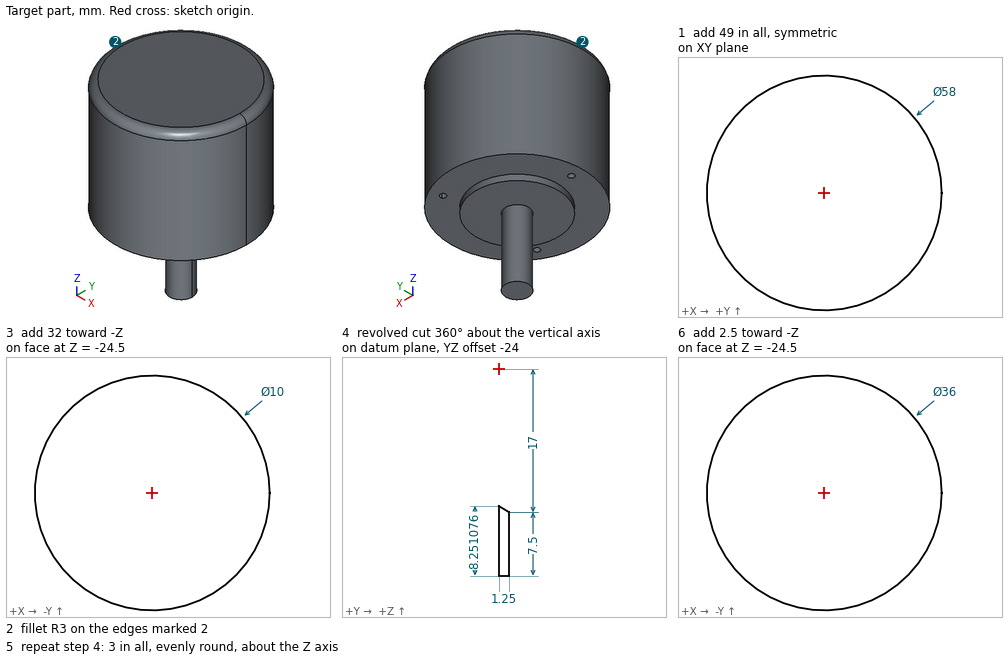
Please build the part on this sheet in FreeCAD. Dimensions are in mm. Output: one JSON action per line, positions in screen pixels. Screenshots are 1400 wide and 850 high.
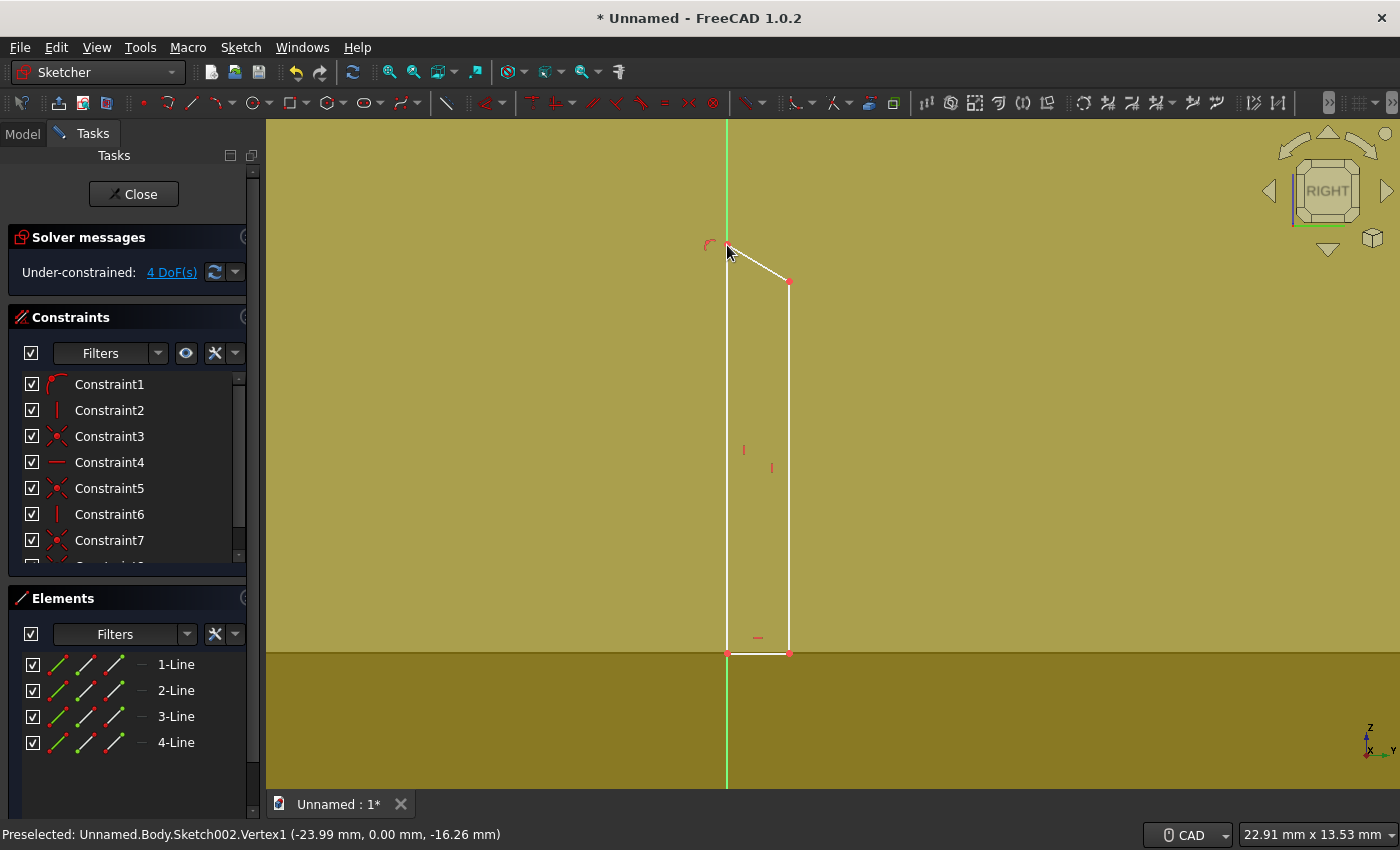
{"action": "left_click", "coordinate": [486, 104]}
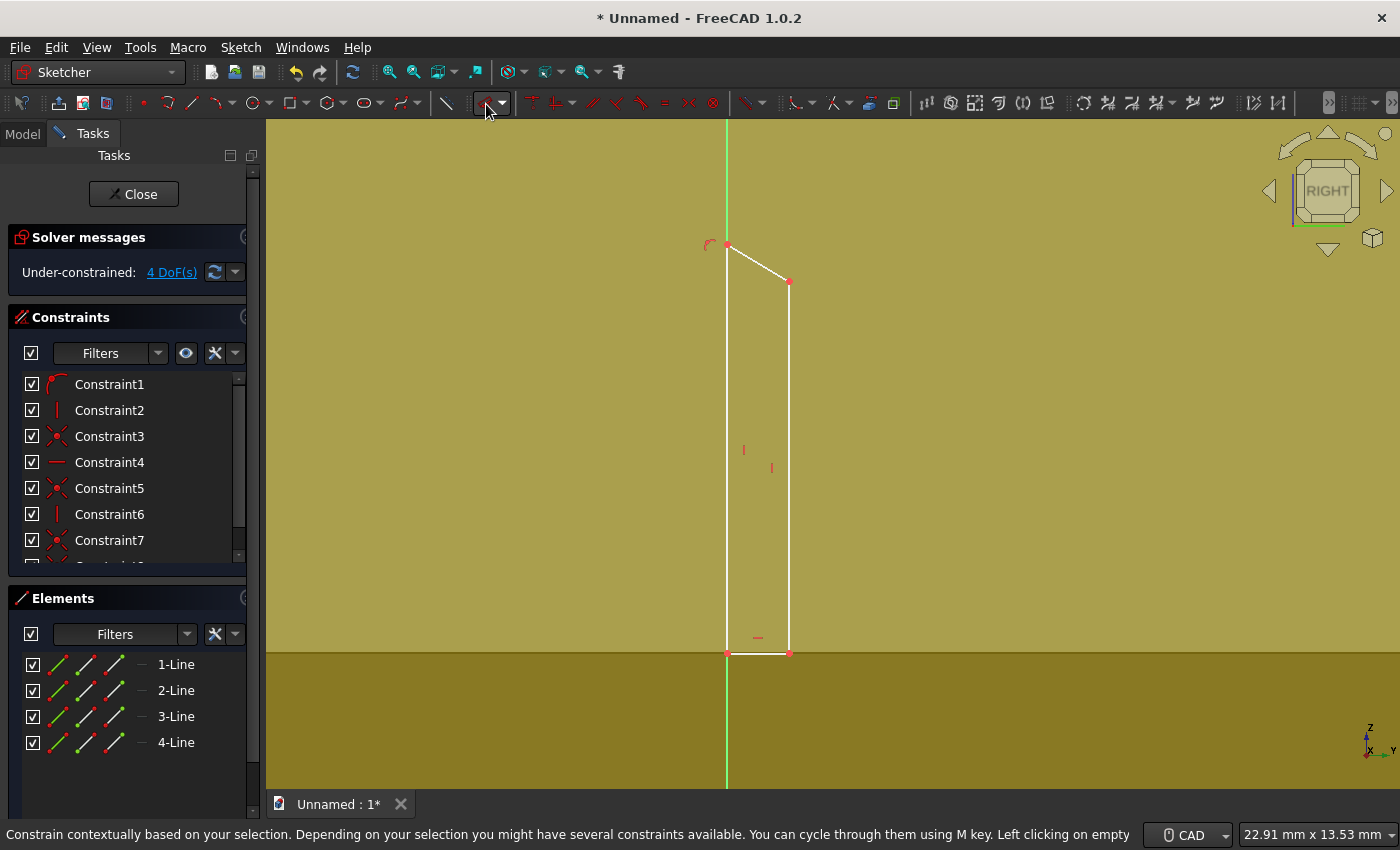
{"action": "left_click", "coordinate": [789, 542]}
{"action": "left_click", "coordinate": [823, 468]}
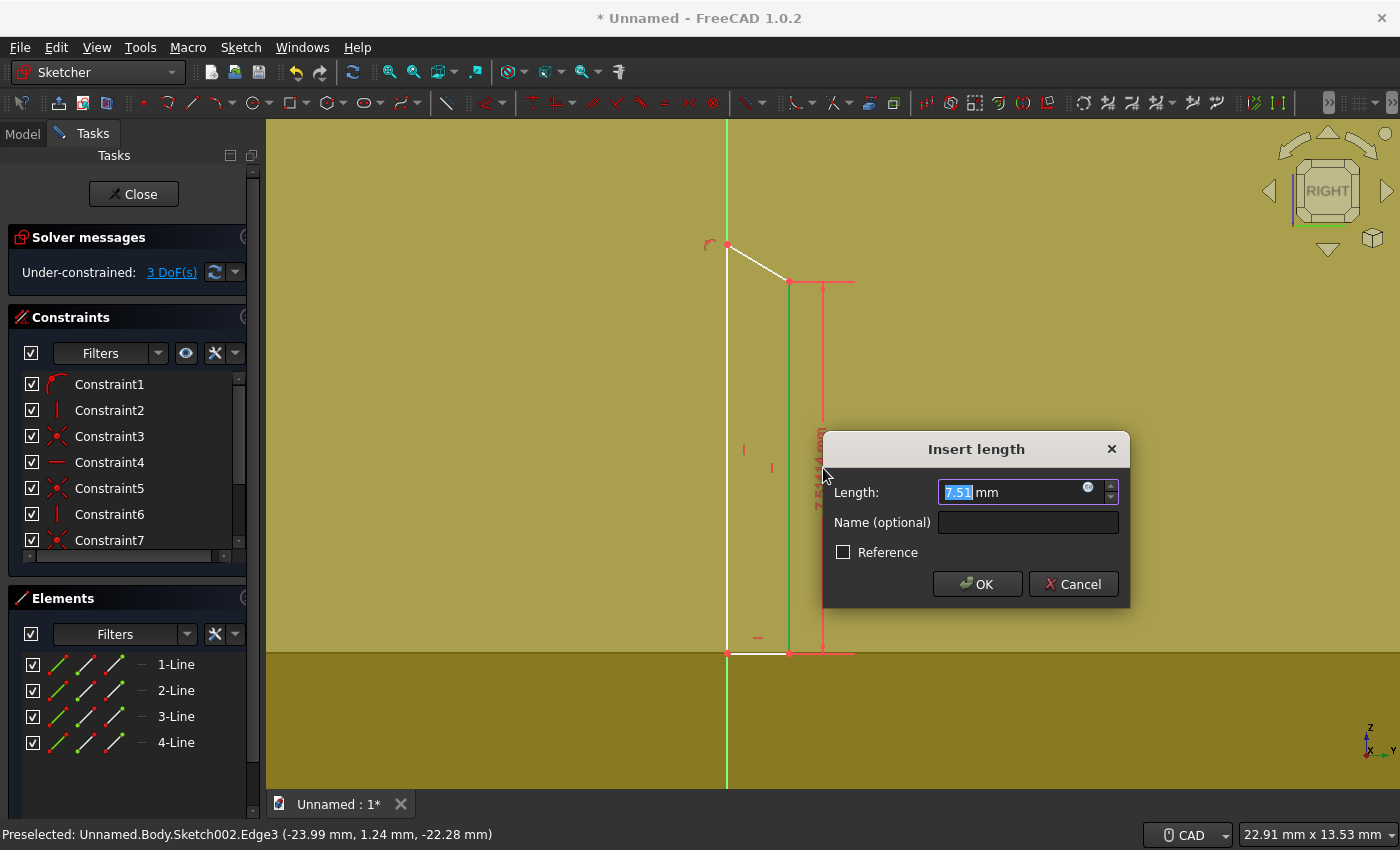
{"action": "type", "text": "7.5"}
{"action": "key", "text": "Return"}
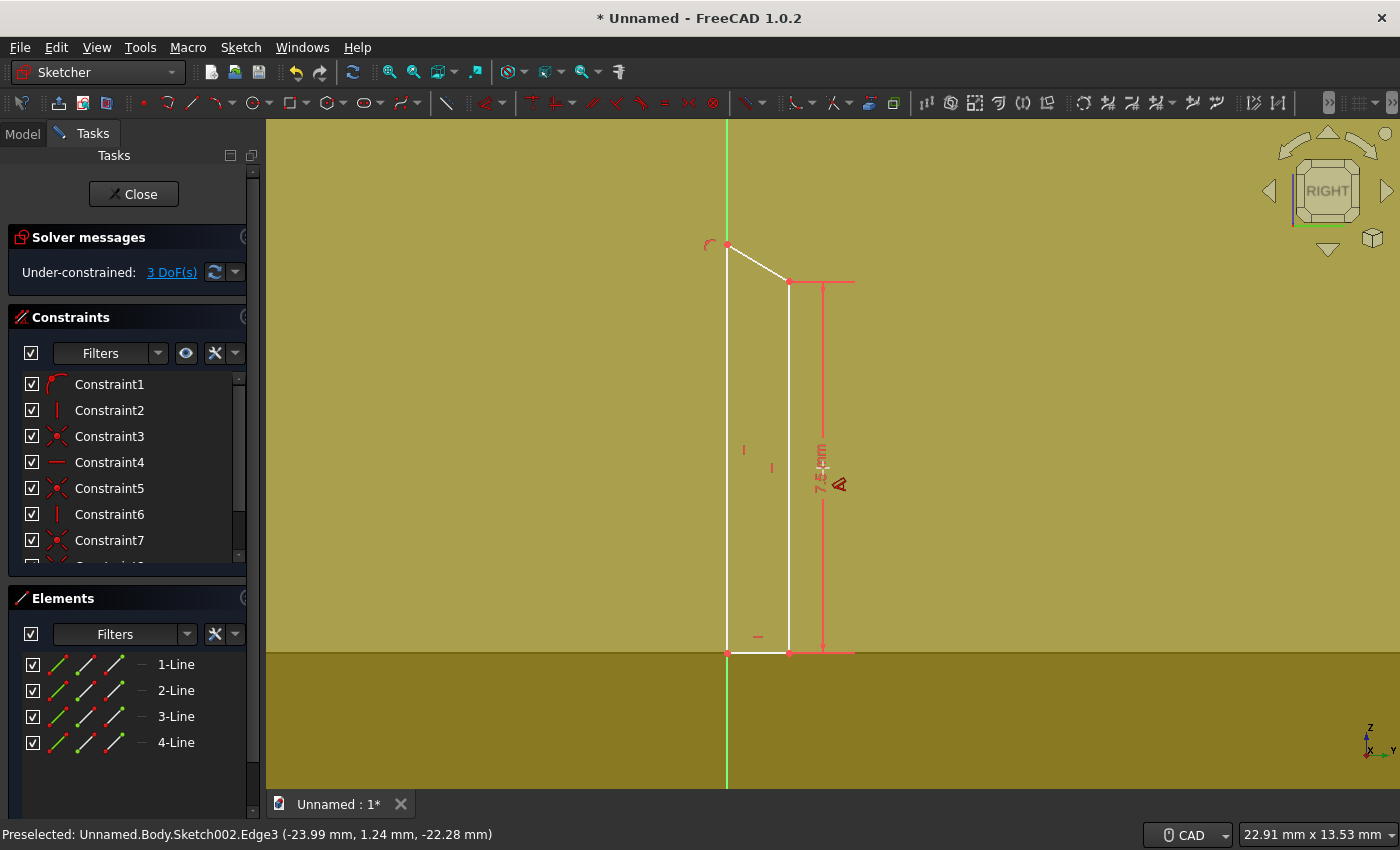
{"action": "left_click", "coordinate": [789, 282]}
{"action": "left_click", "coordinate": [693, 215]}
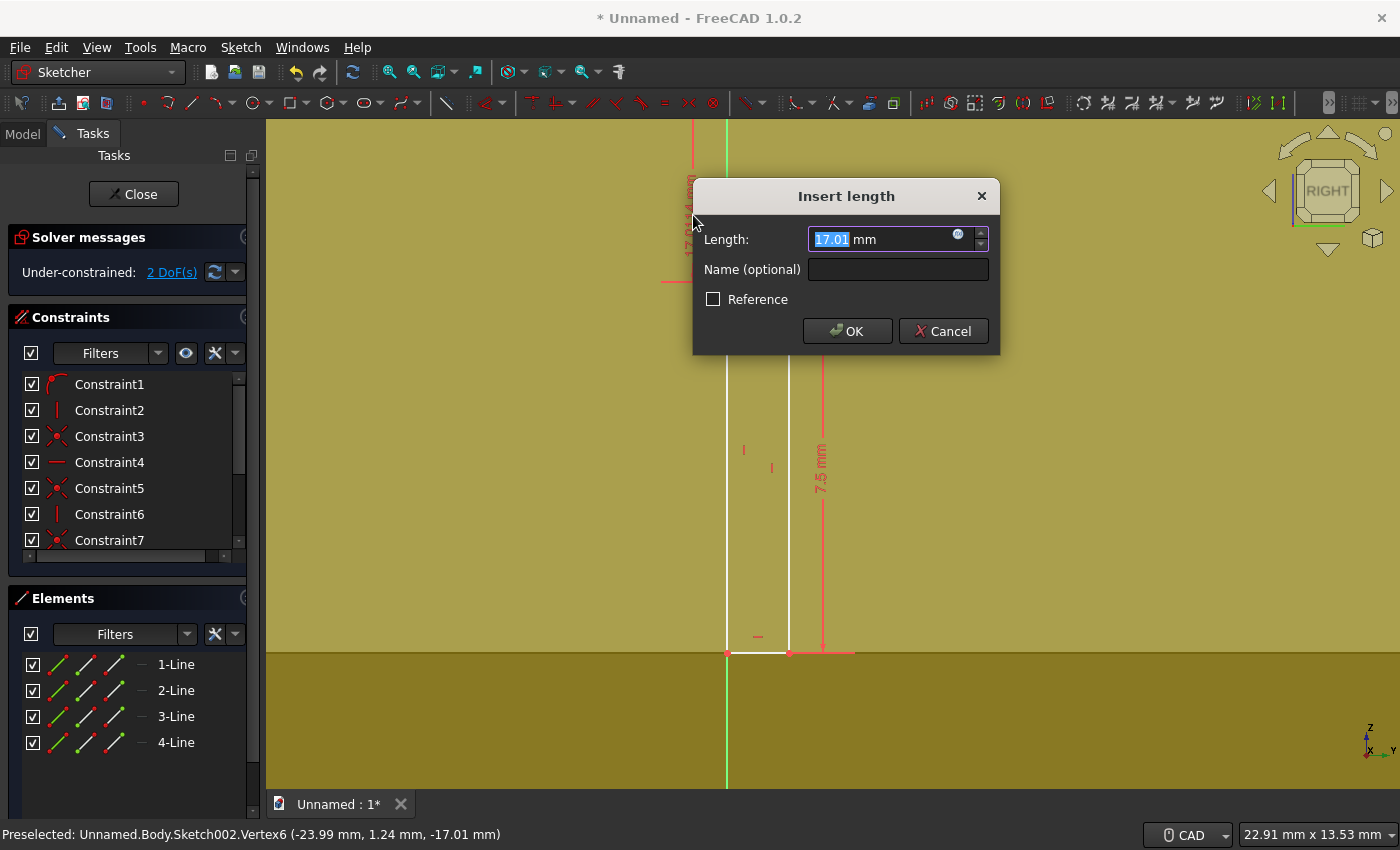
{"action": "type", "text": "17"}
{"action": "key", "text": "Return"}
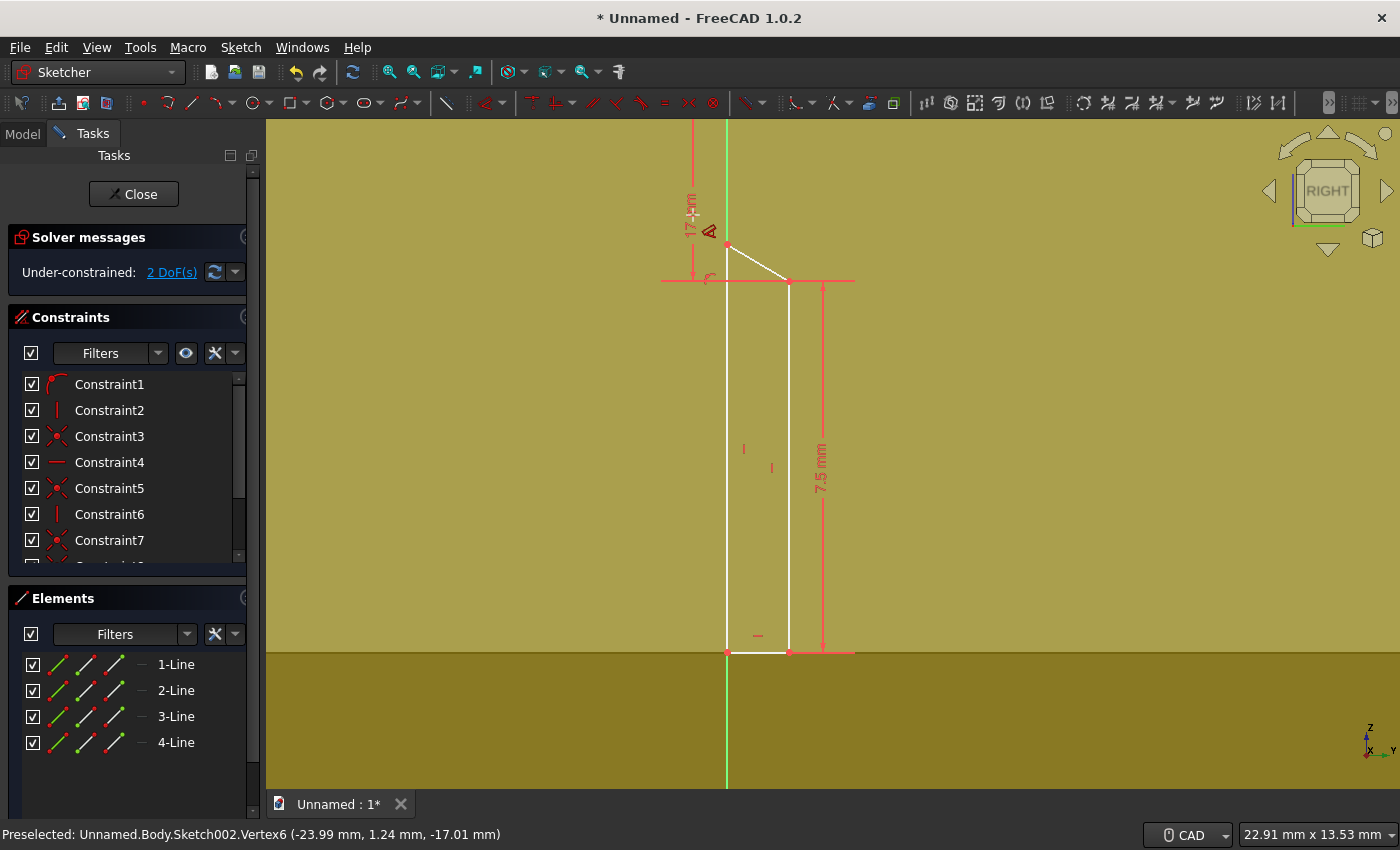
{"action": "left_click", "coordinate": [746, 653]}
{"action": "left_click", "coordinate": [758, 687]}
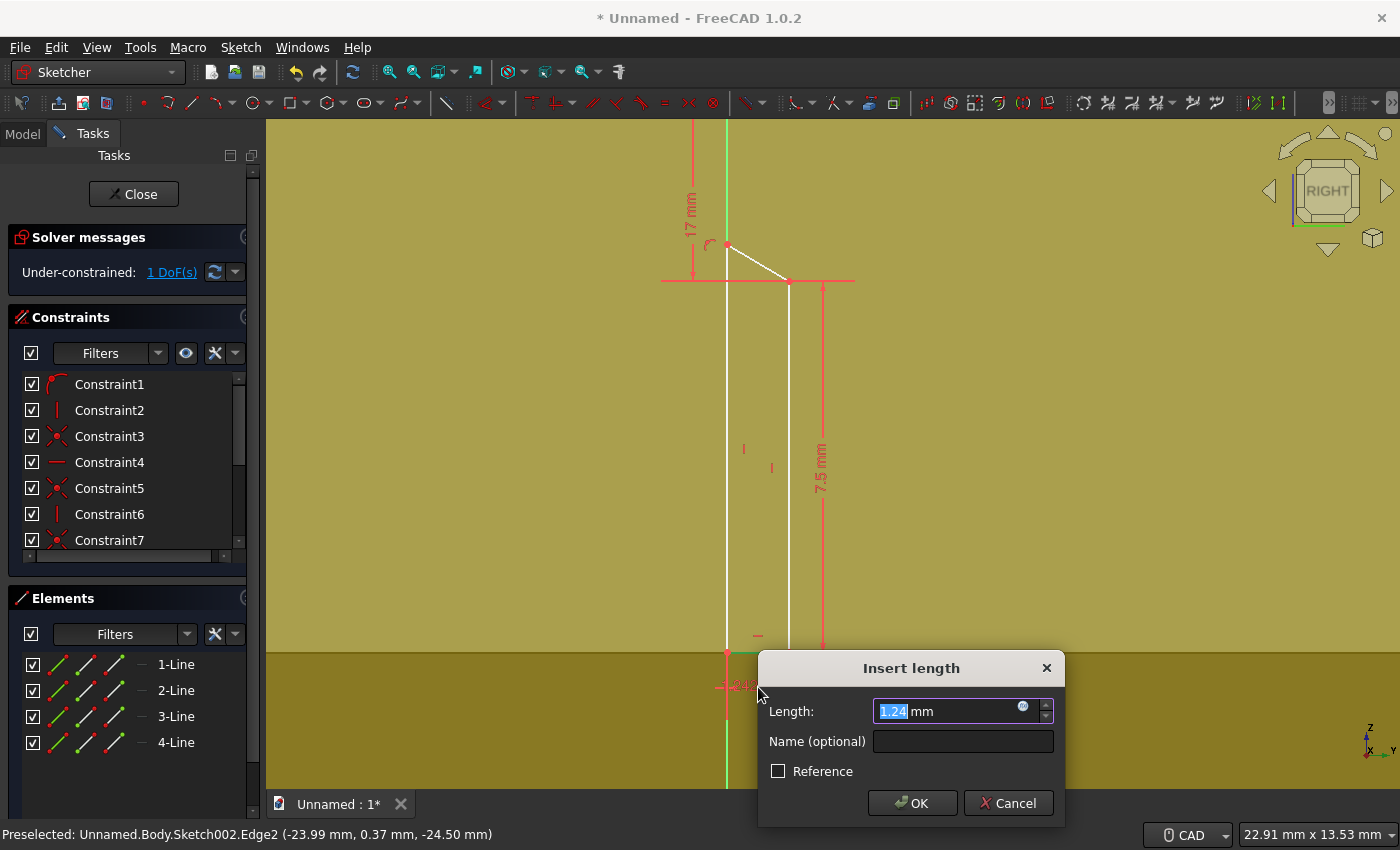
{"action": "type", "text": "1.25"}
{"action": "key", "text": "Return"}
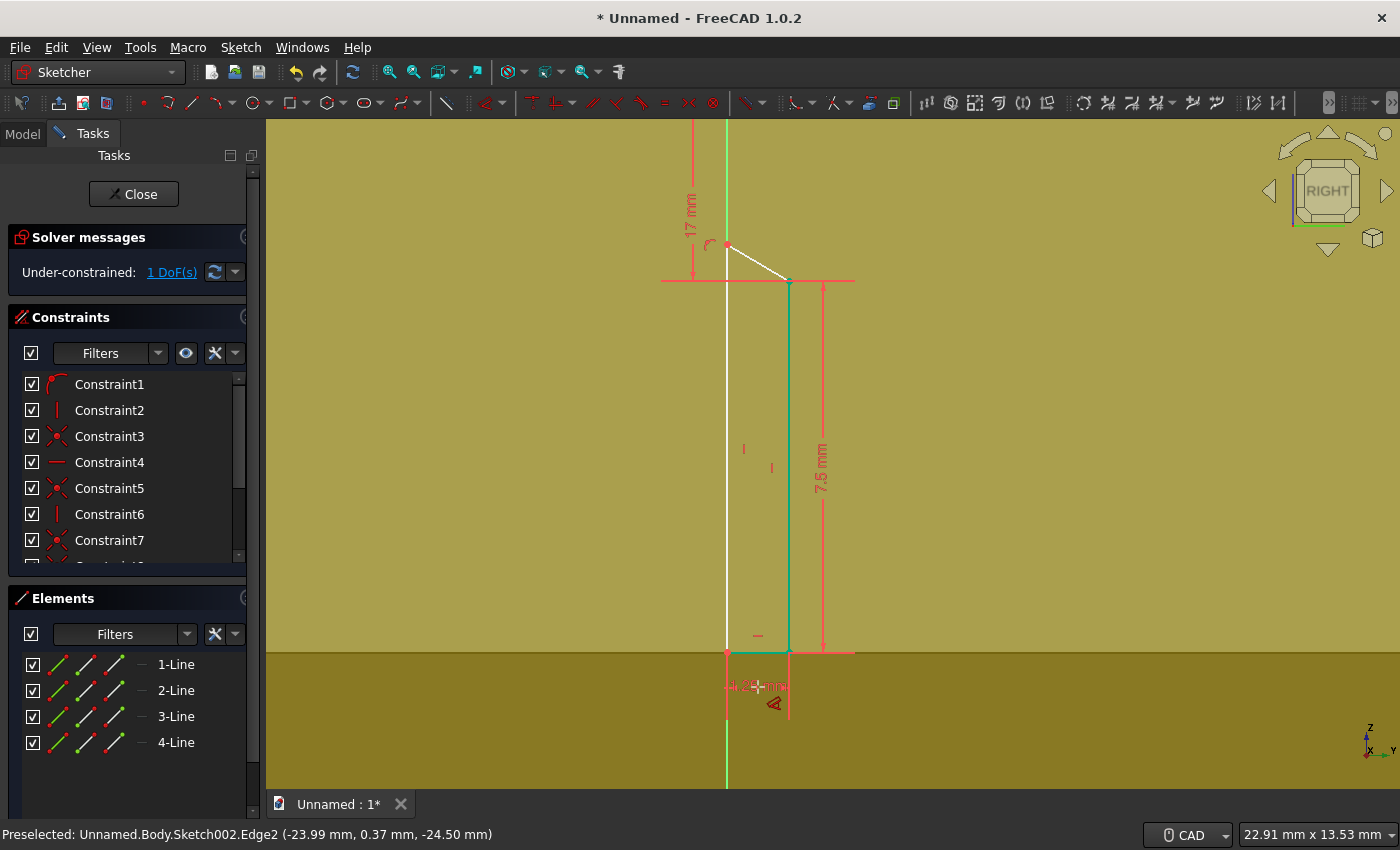
{"action": "left_click", "coordinate": [727, 367]}
{"action": "left_click", "coordinate": [693, 449]}